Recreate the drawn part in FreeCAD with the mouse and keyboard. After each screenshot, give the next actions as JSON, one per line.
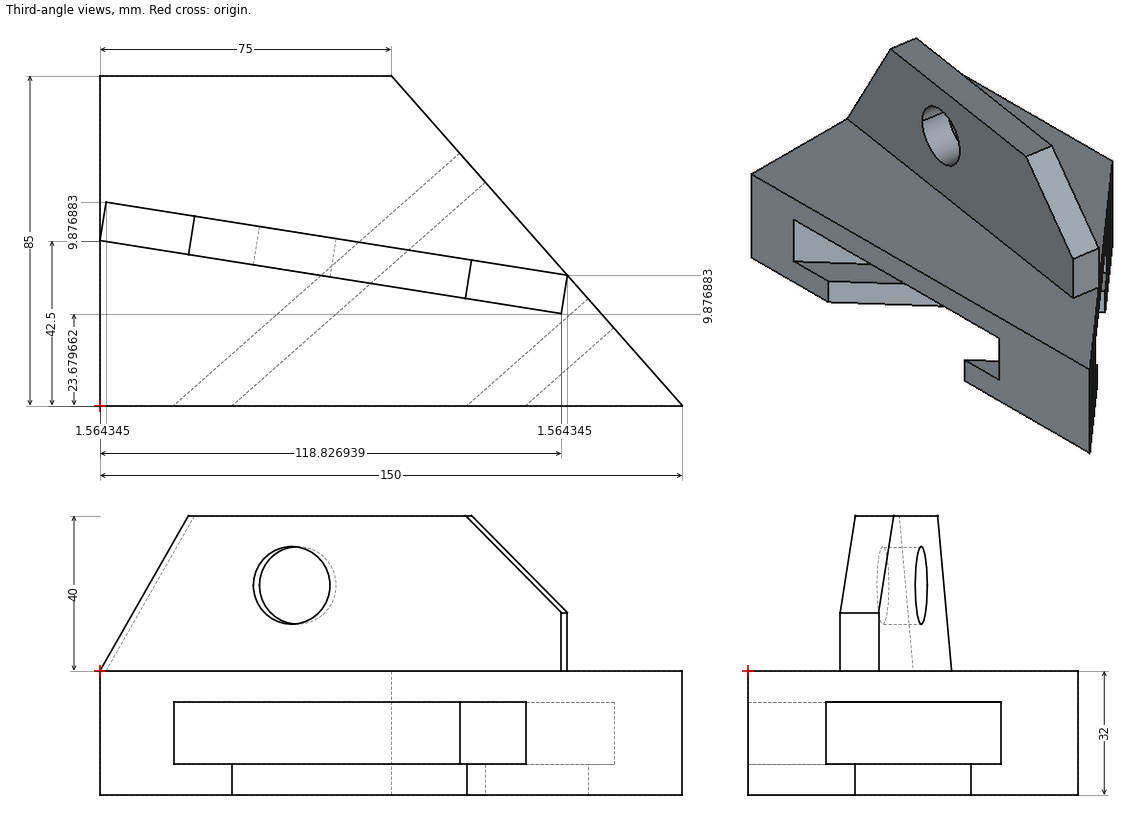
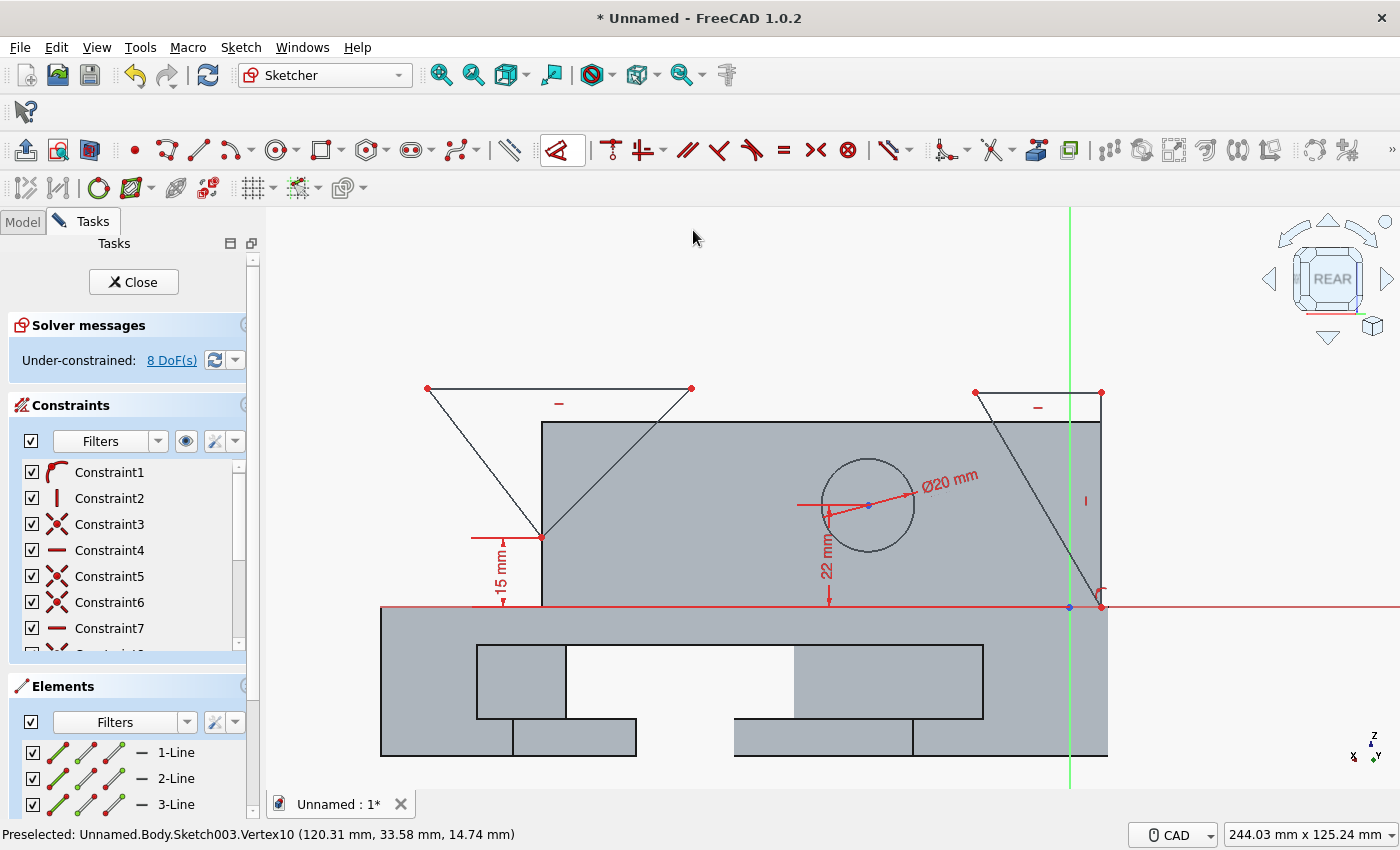
{"action": "left_click", "coordinate": [1101, 607]}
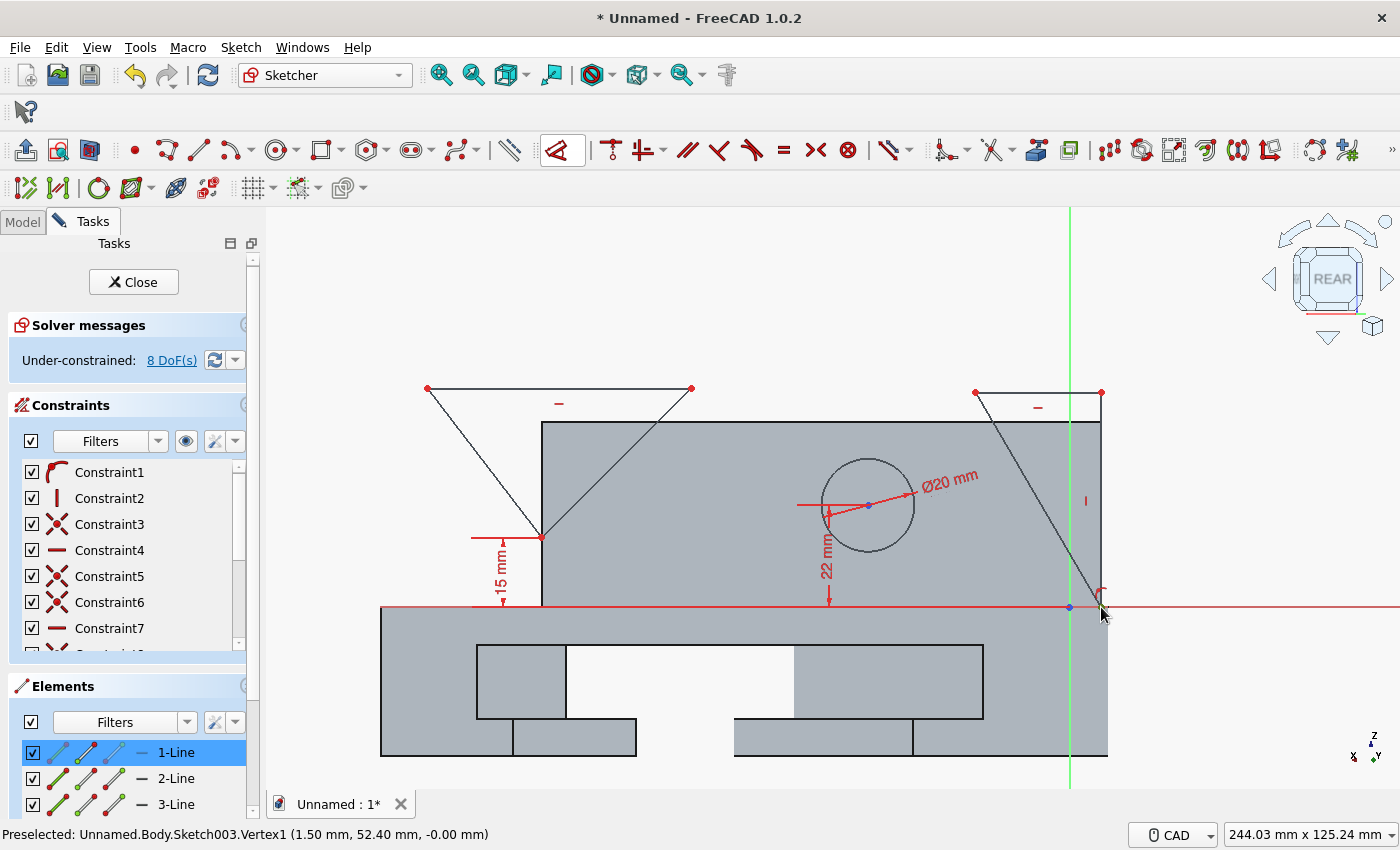
{"action": "left_click", "coordinate": [868, 505]}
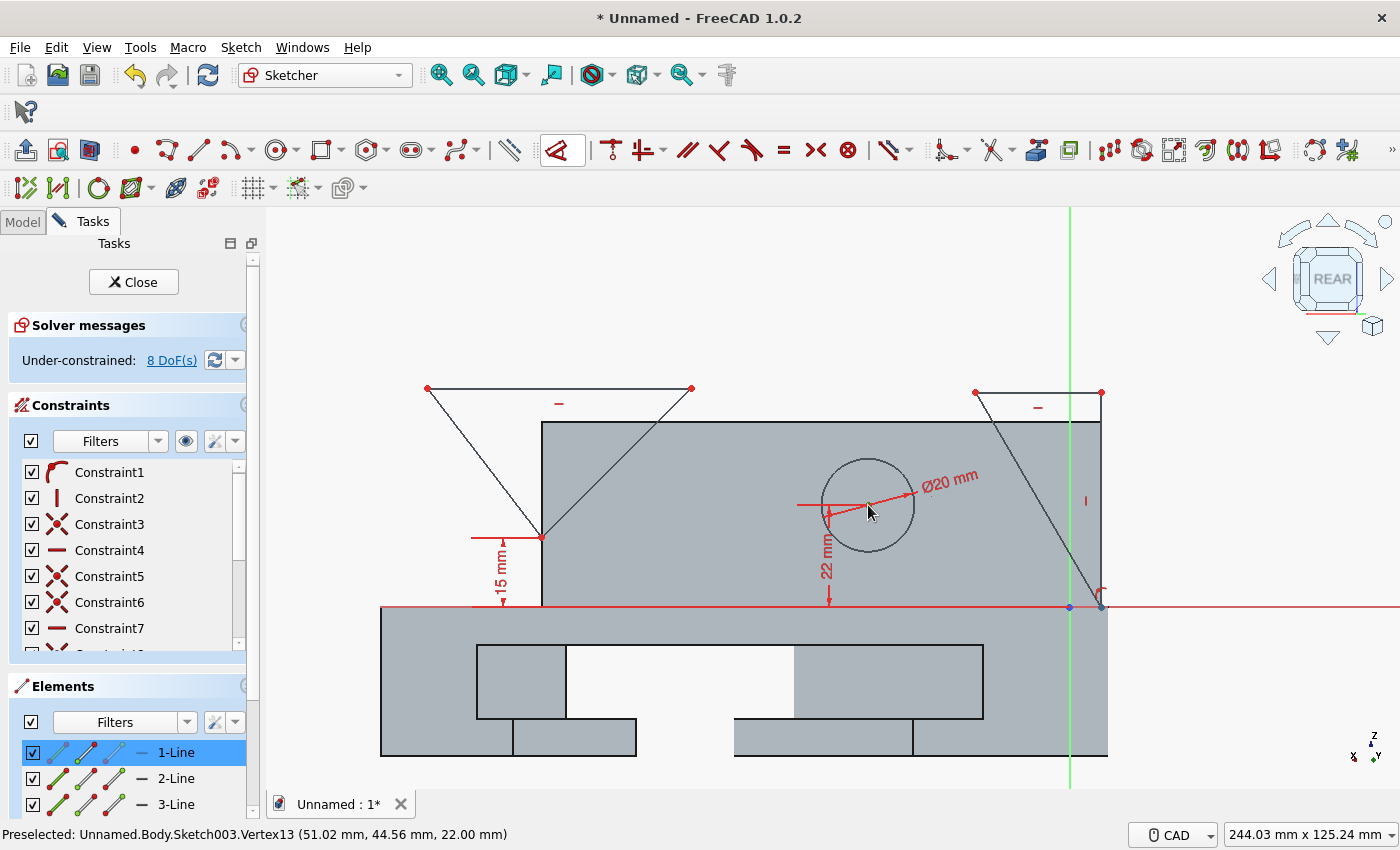
{"action": "key", "text": "l"}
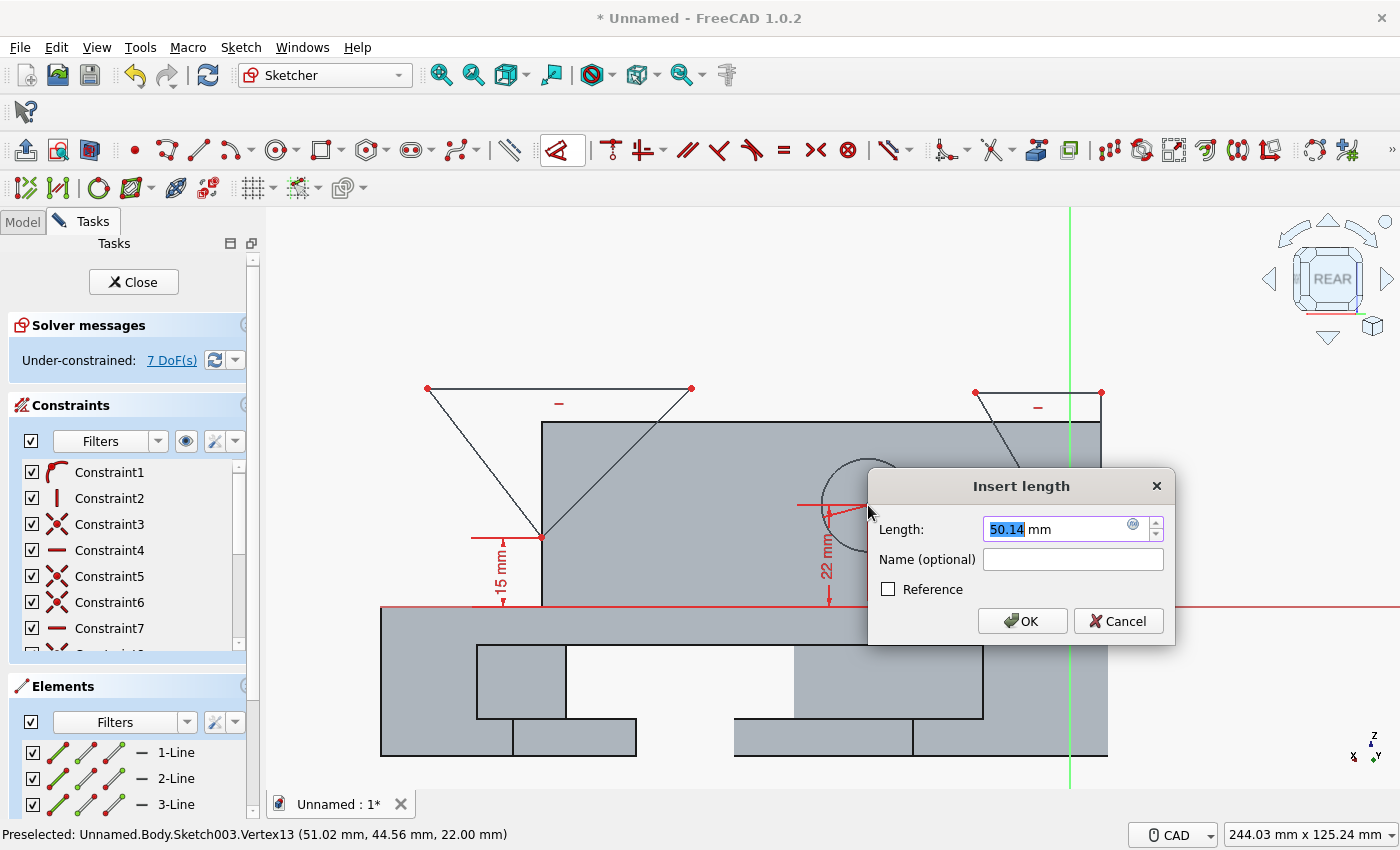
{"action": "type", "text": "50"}
{"action": "key", "text": "Return"}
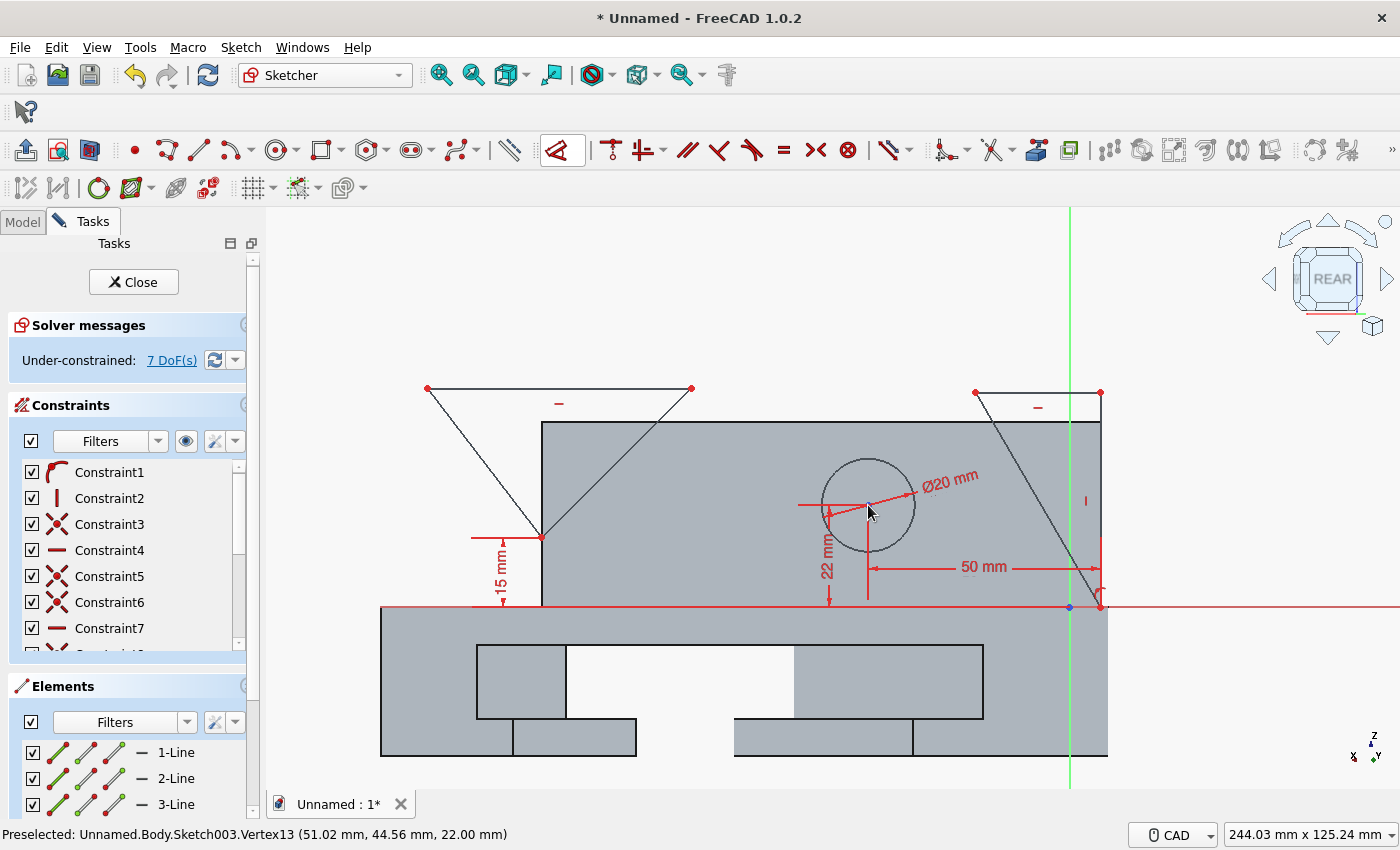
{"action": "left_click", "coordinate": [1101, 543]}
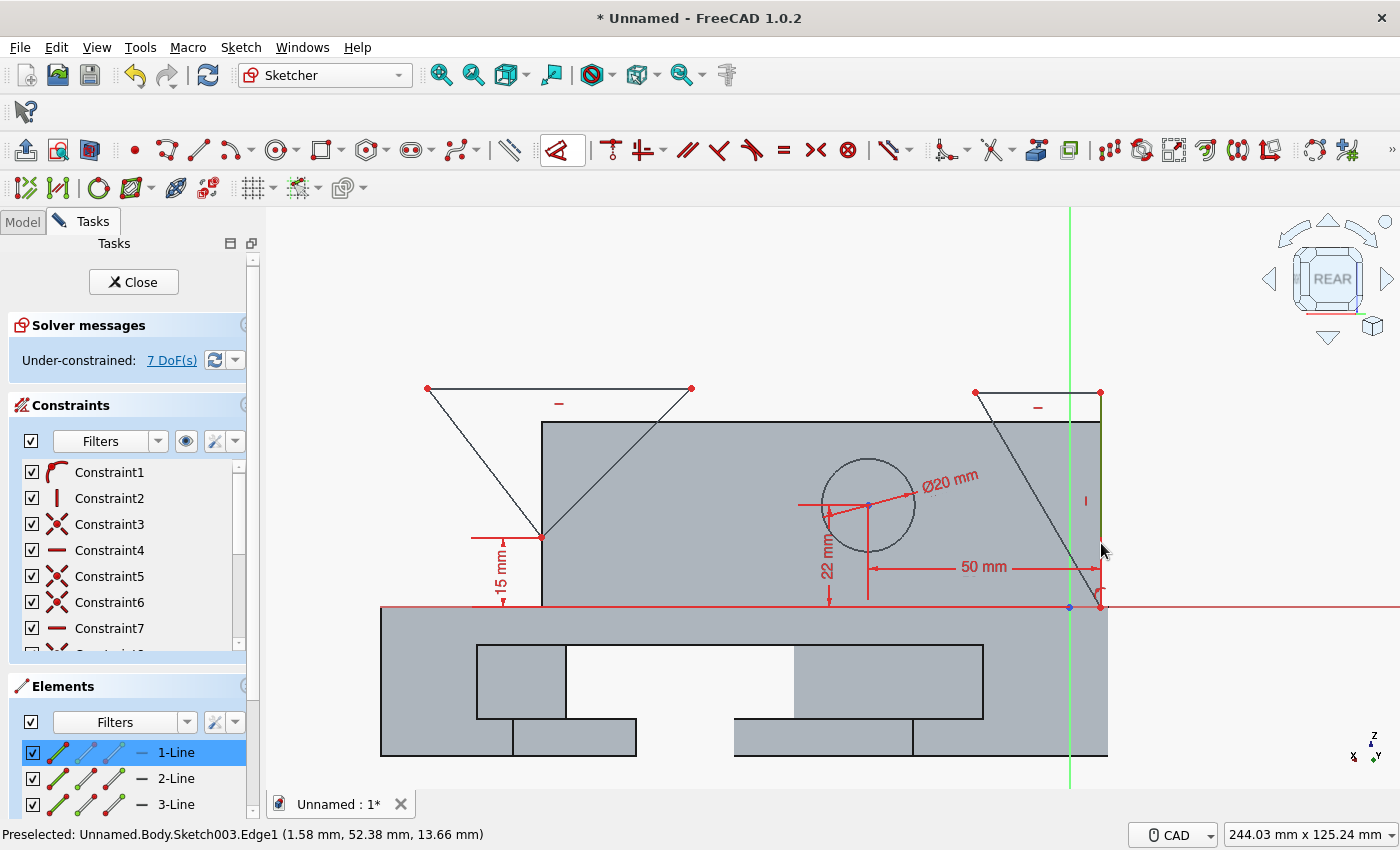
{"action": "key", "text": "i"}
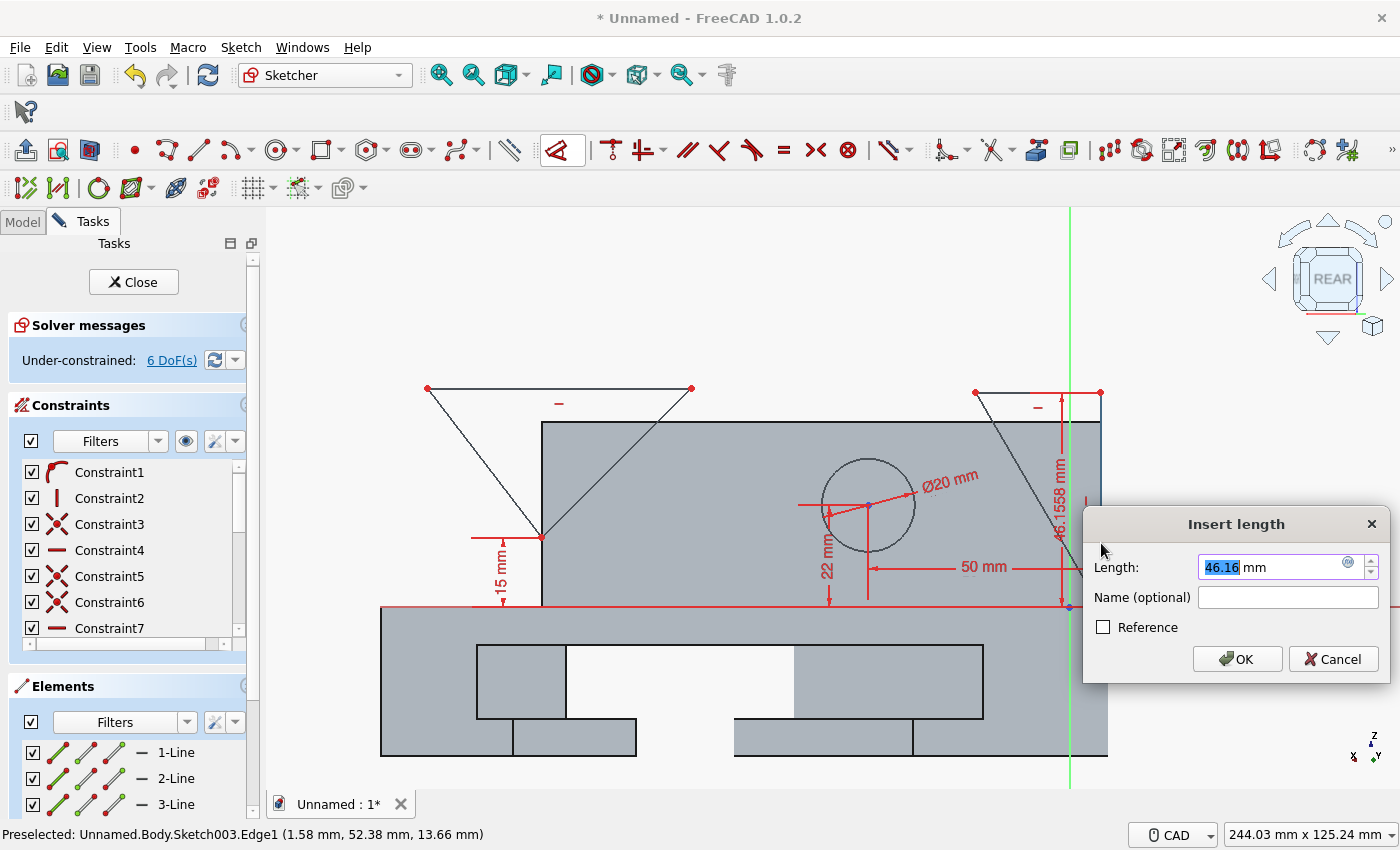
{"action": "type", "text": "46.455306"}
{"action": "key", "text": "Return"}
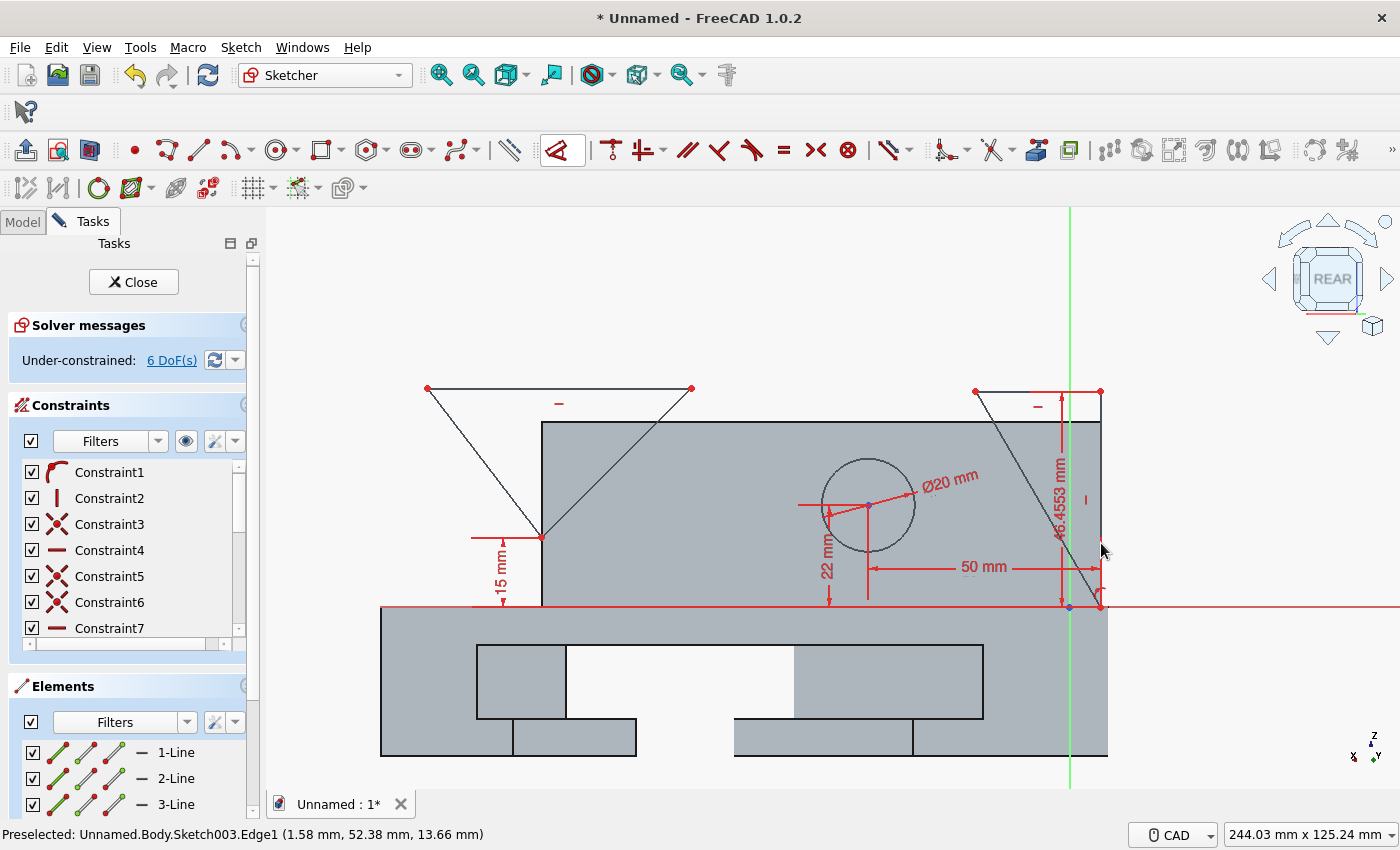
{"action": "left_click", "coordinate": [1013, 392]}